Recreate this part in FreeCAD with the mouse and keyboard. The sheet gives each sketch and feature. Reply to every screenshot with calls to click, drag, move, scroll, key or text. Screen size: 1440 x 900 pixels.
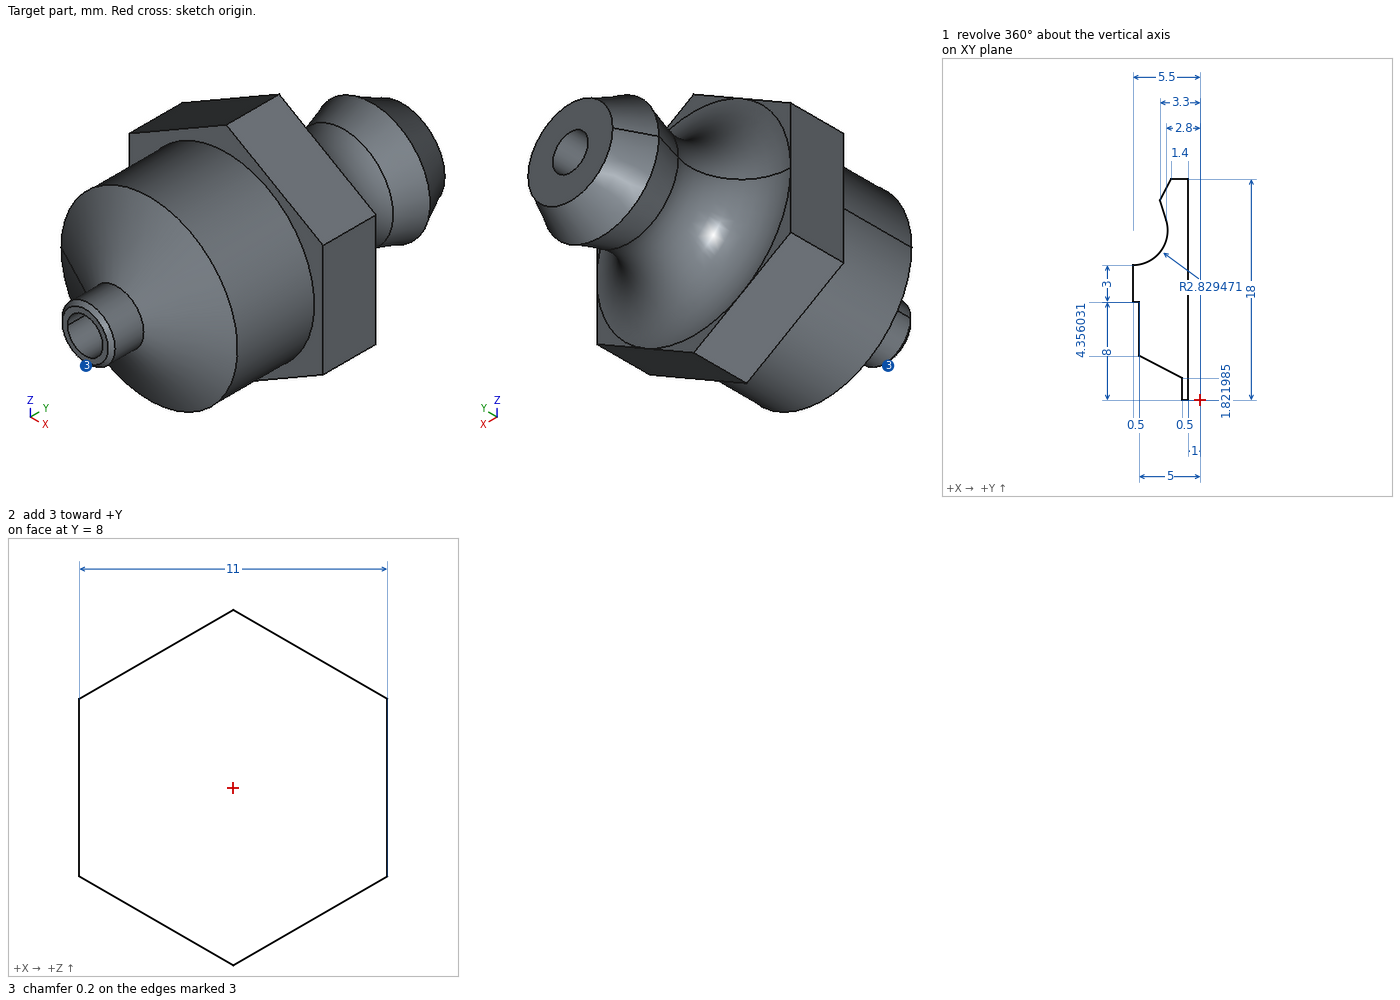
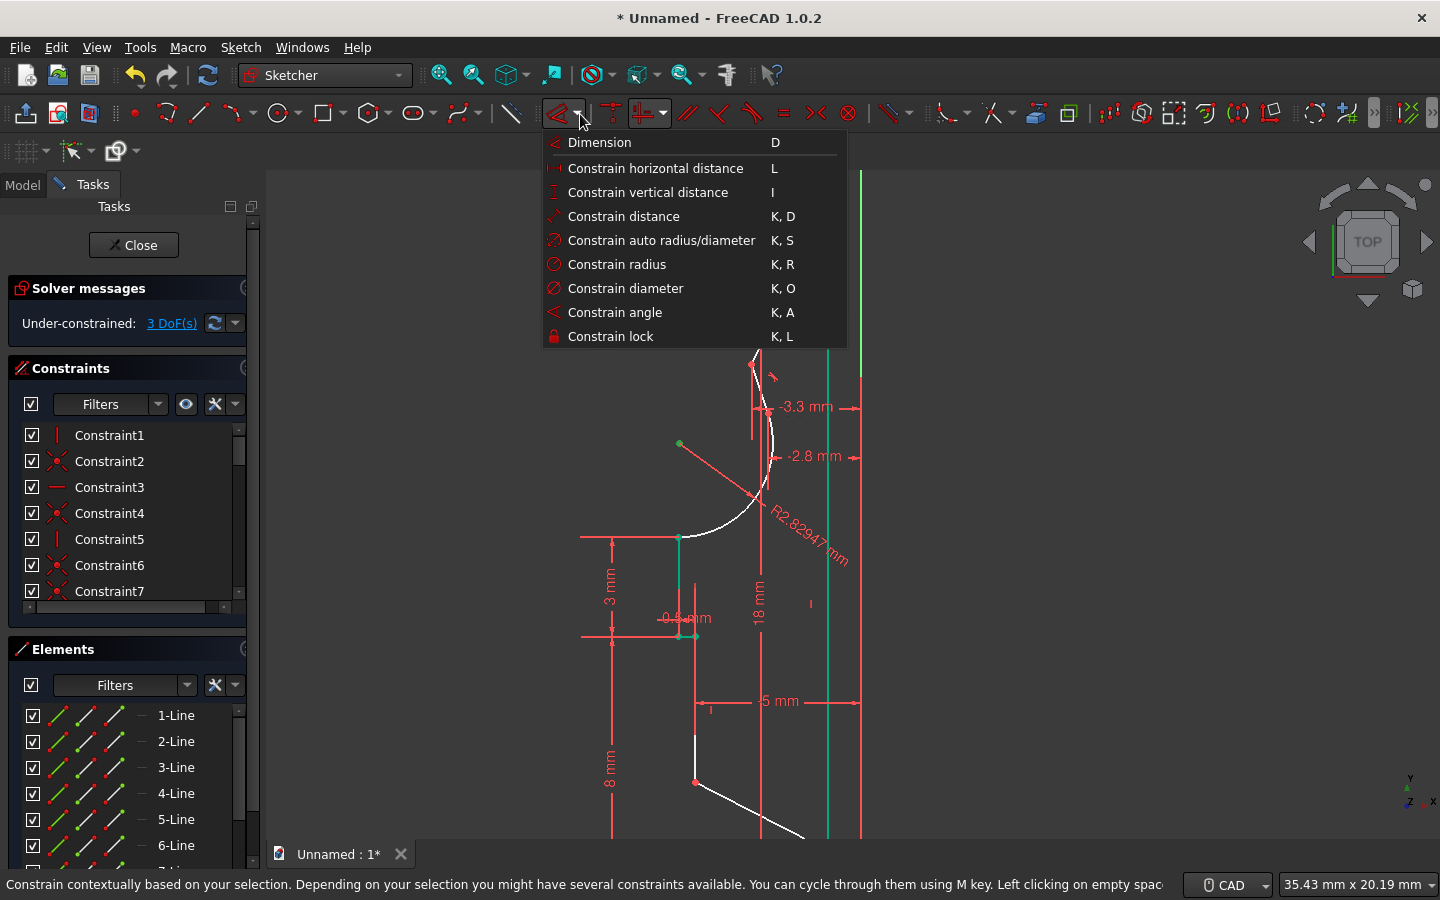
click(695, 168)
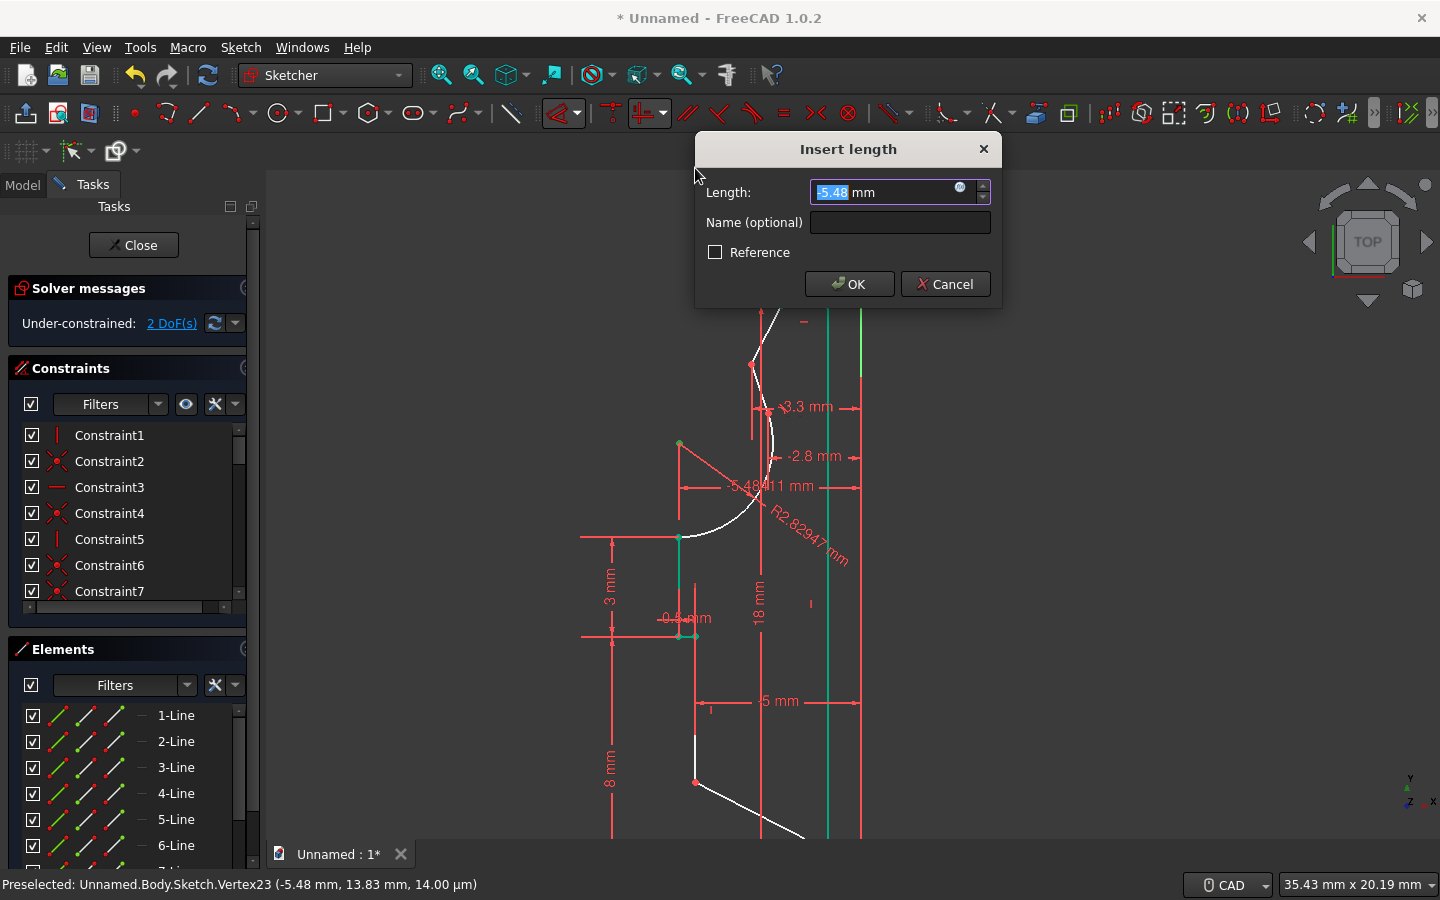
text(-5.5)
key(Return)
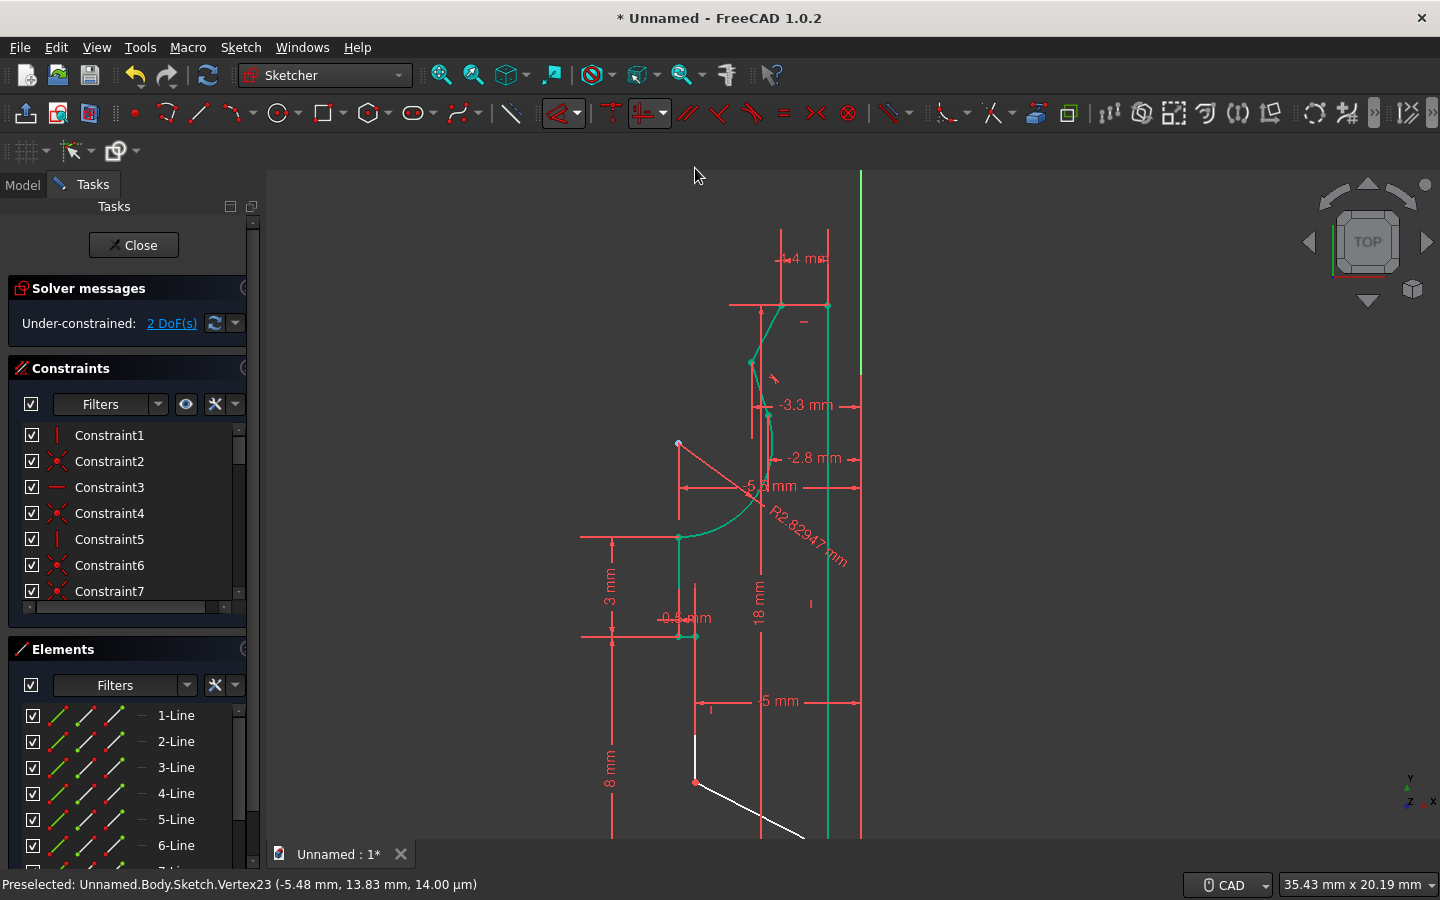
click(695, 680)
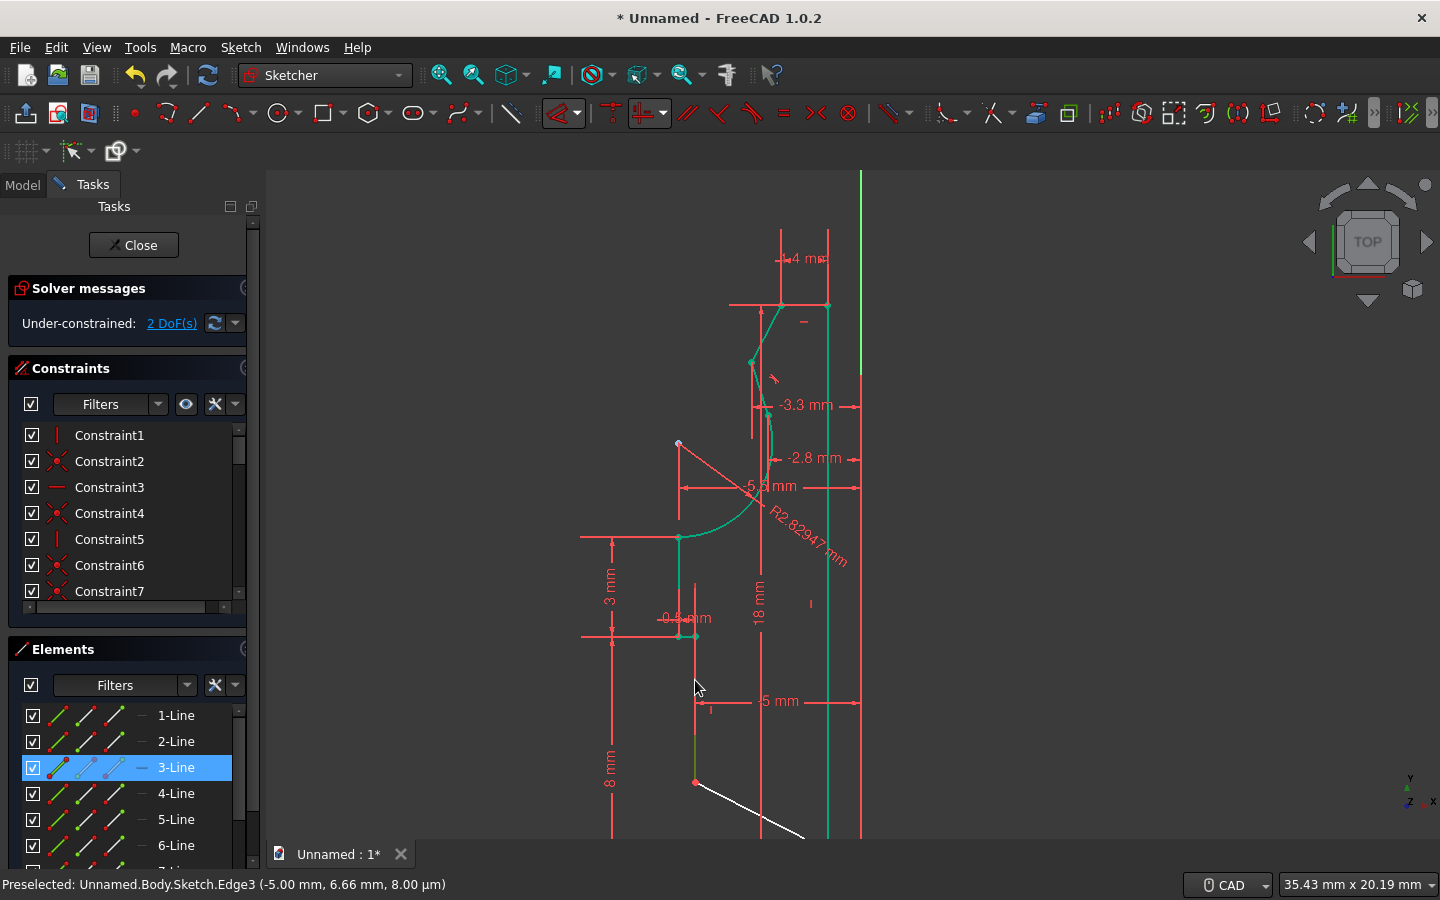
click(580, 114)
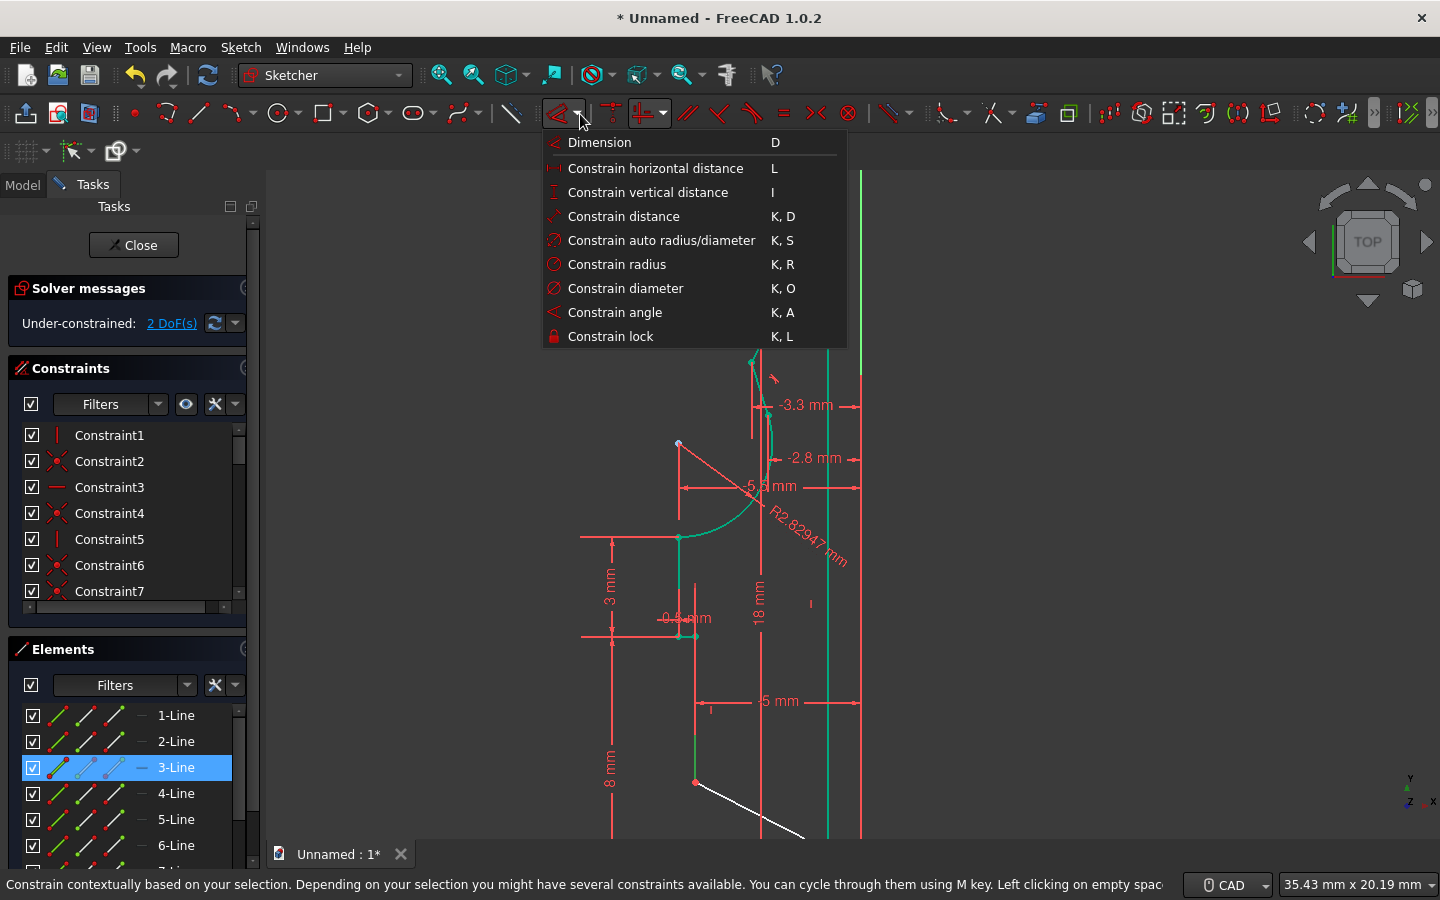
click(695, 192)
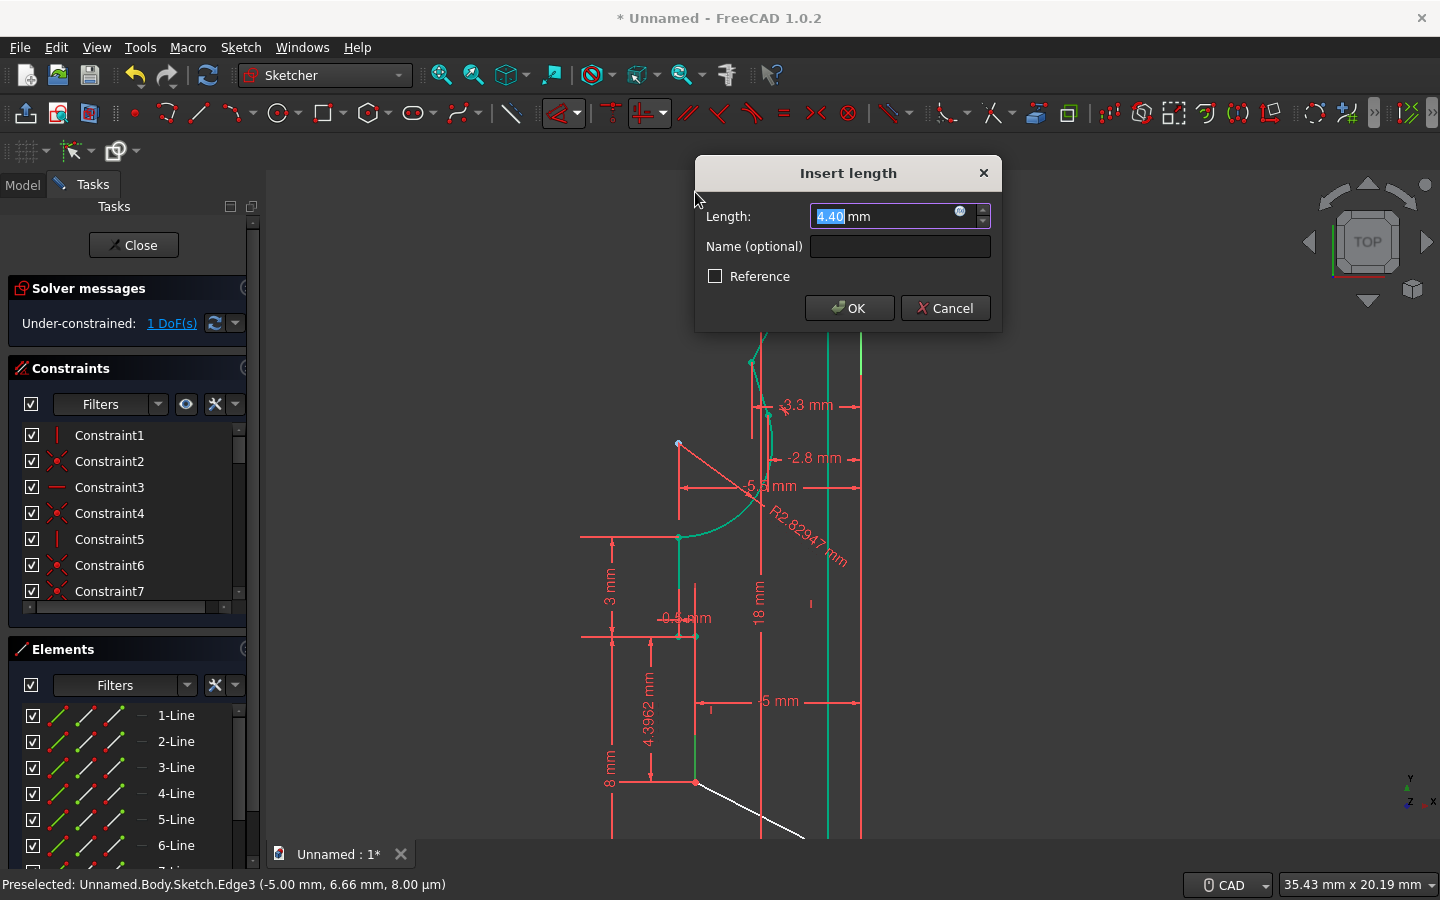
text(4.356031)
key(Return)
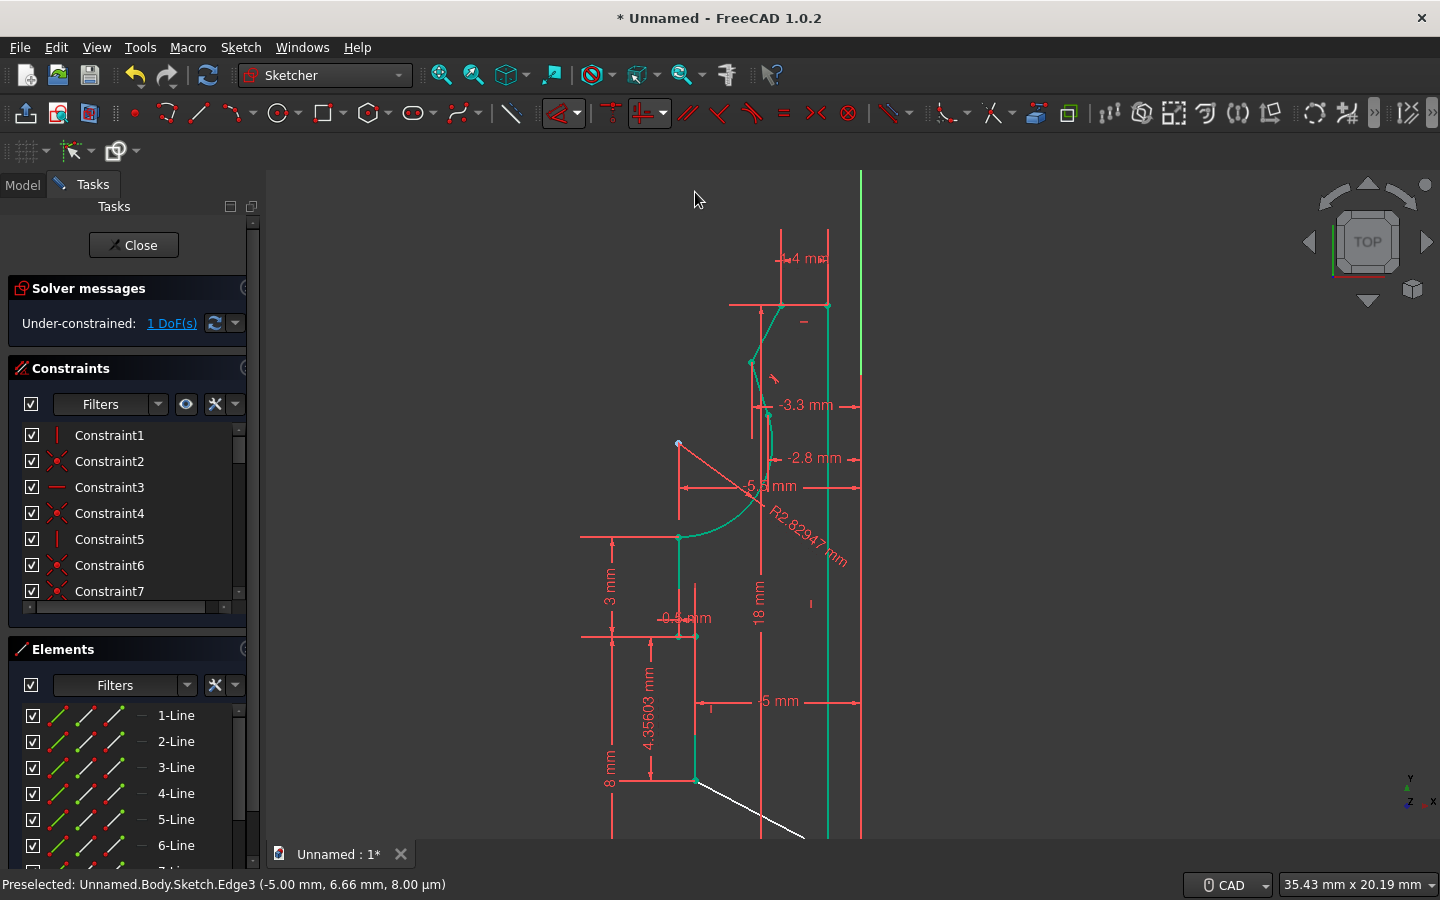
scroll(814, 303, down, 2)